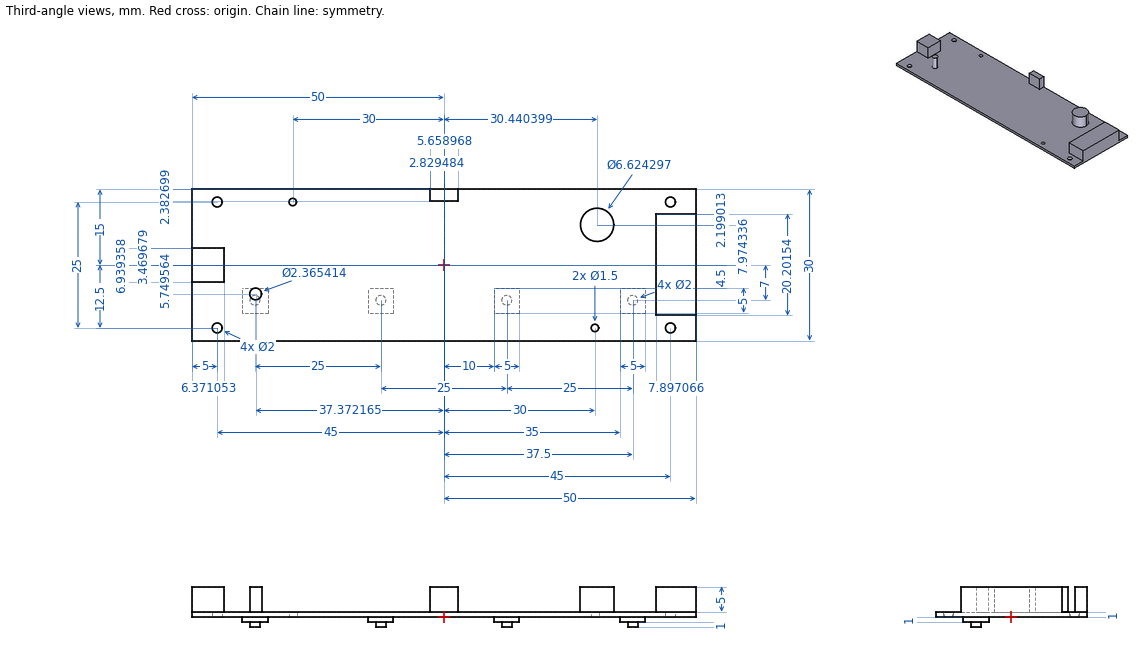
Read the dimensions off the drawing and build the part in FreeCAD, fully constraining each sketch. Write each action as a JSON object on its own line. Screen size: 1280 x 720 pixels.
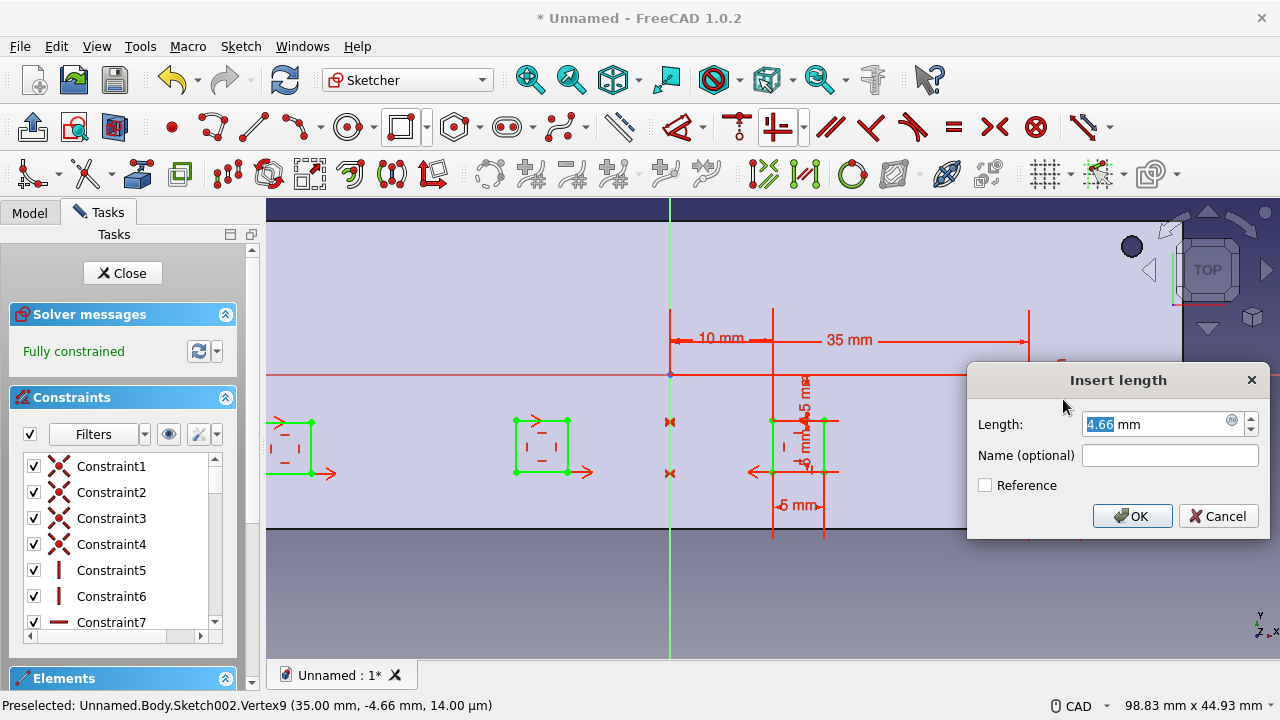
{"action": "type", "text": "4.5"}
{"action": "key", "text": "Return"}
{"action": "key", "text": "Escape"}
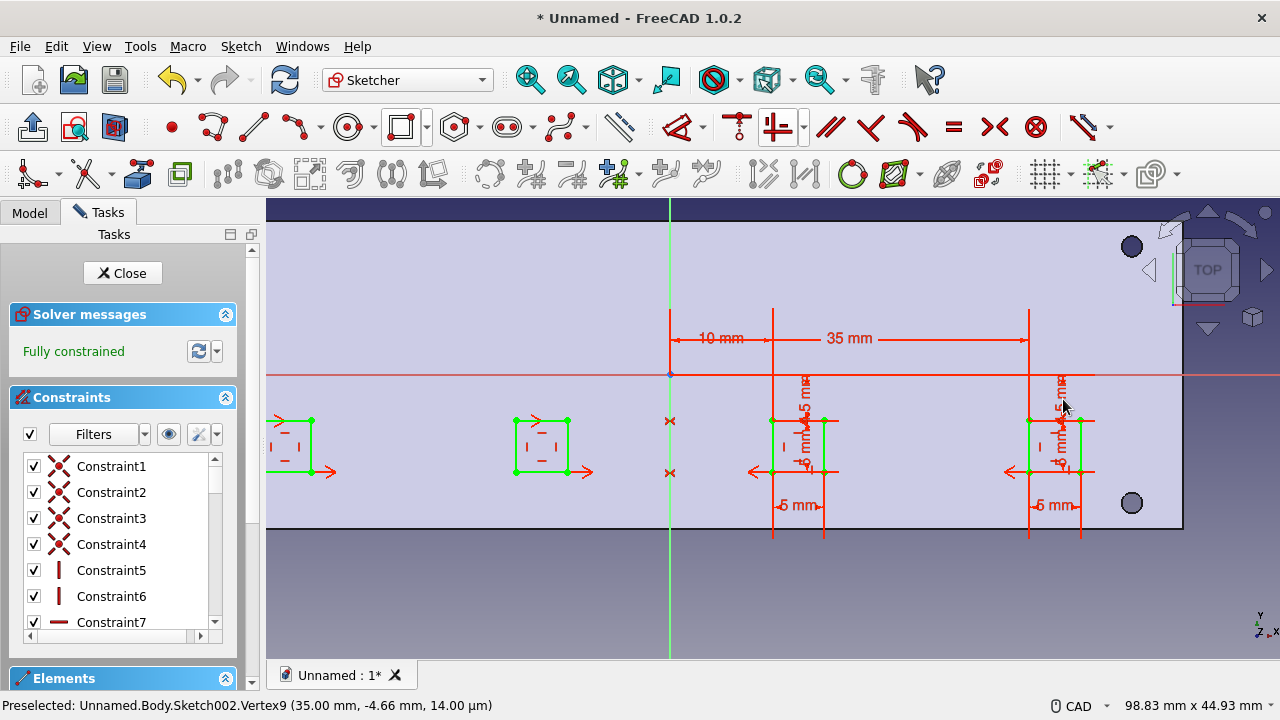
{"action": "left_click", "coordinate": [123, 273]}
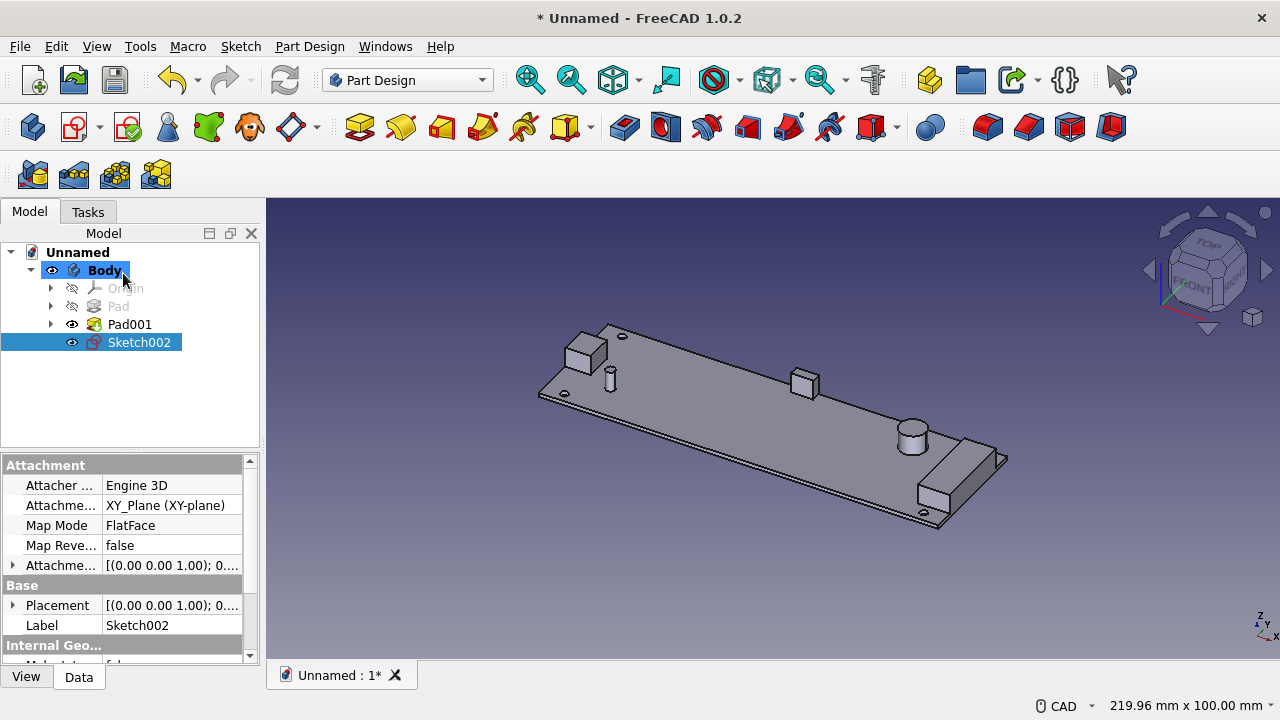
{"action": "left_click", "coordinate": [360, 128]}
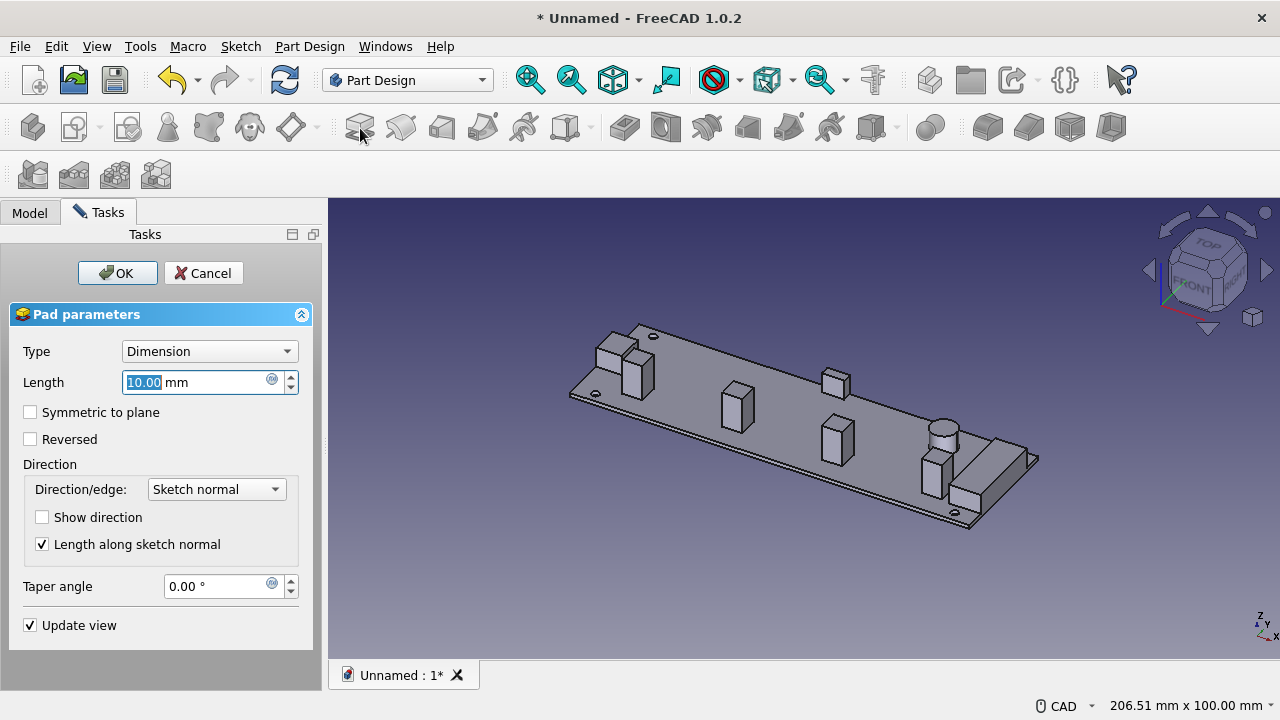
{"action": "type", "text": "1"}
{"action": "key", "text": "Tab"}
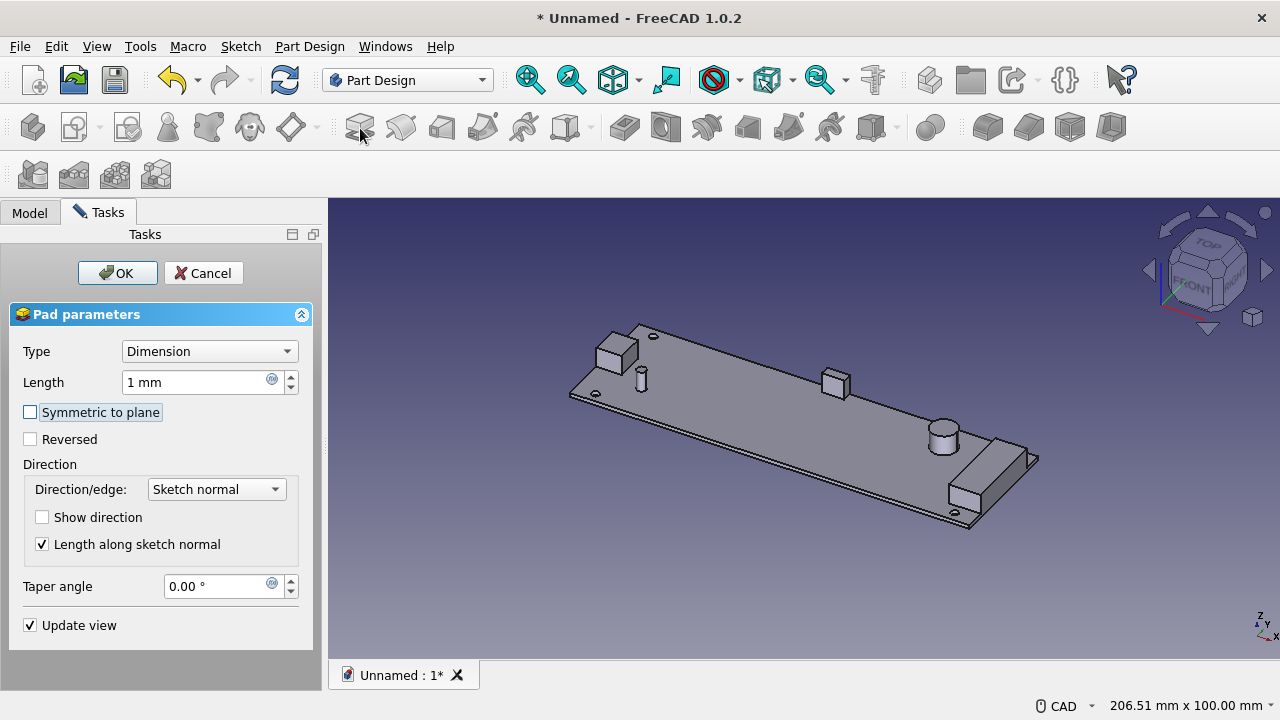
{"action": "left_click", "coordinate": [31, 439]}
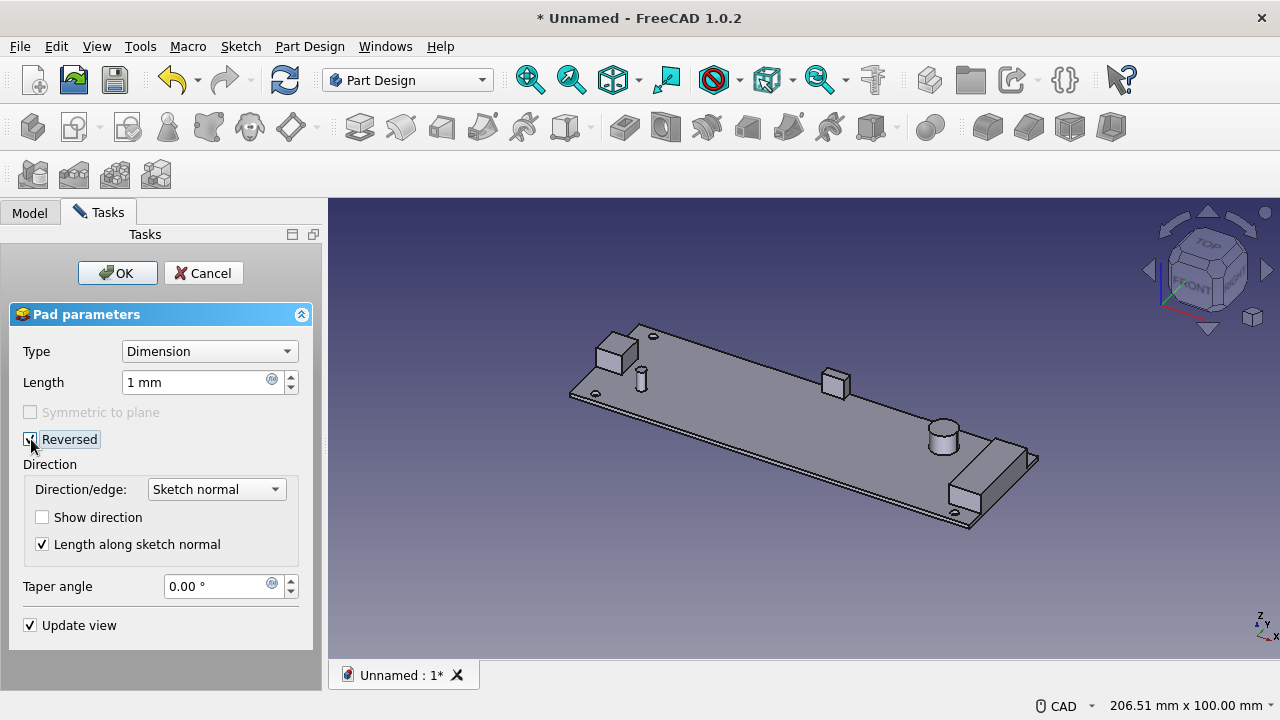
{"action": "left_click", "coordinate": [118, 273]}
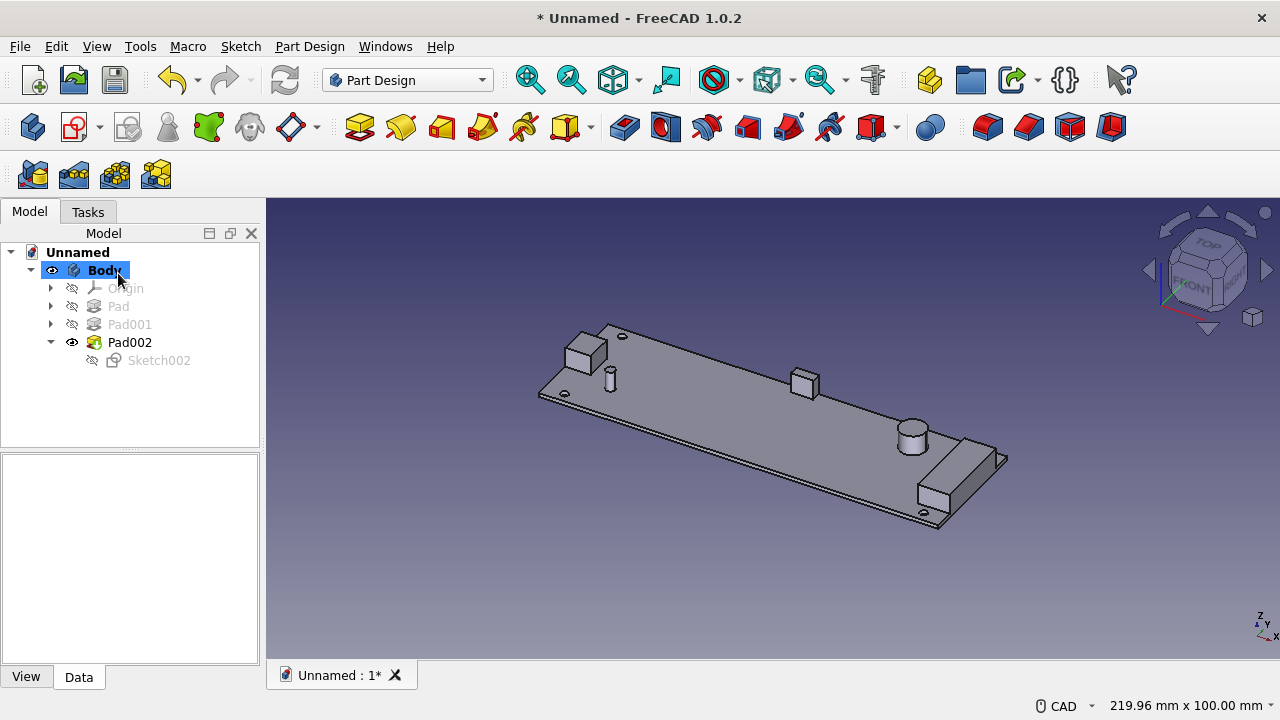
{"action": "key", "text": "5"}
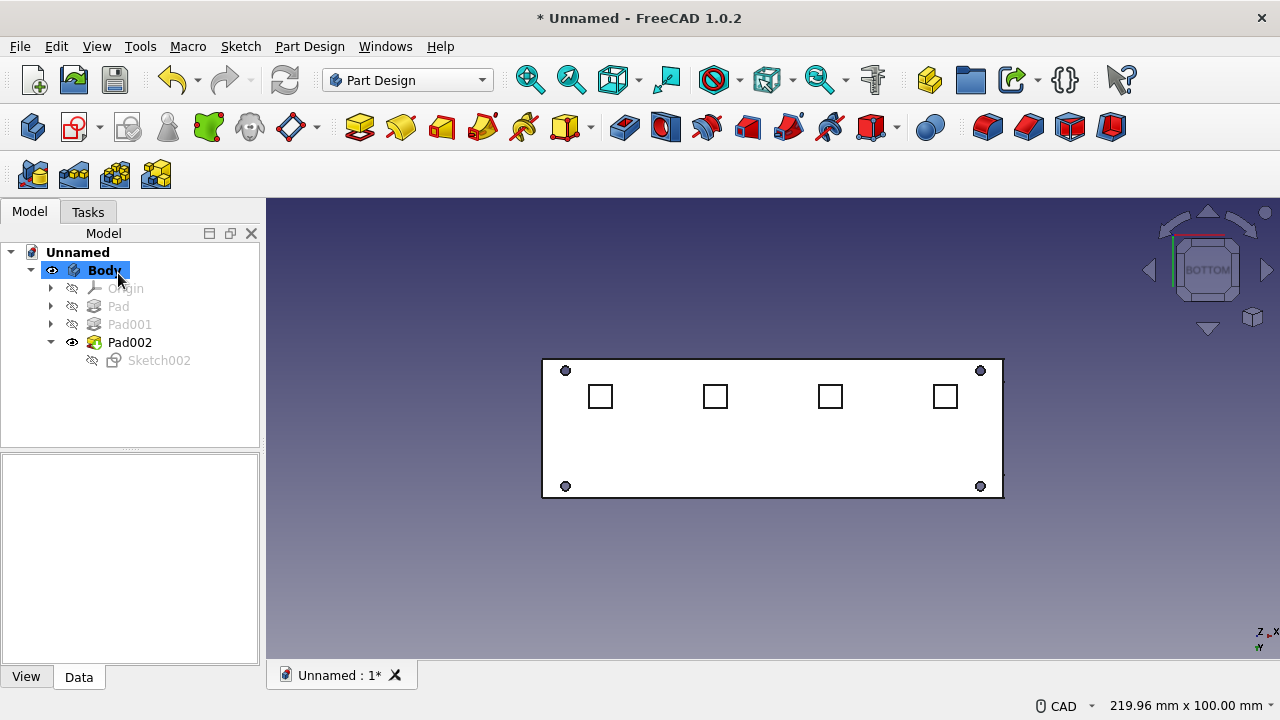
{"action": "left_click", "coordinate": [946, 395]}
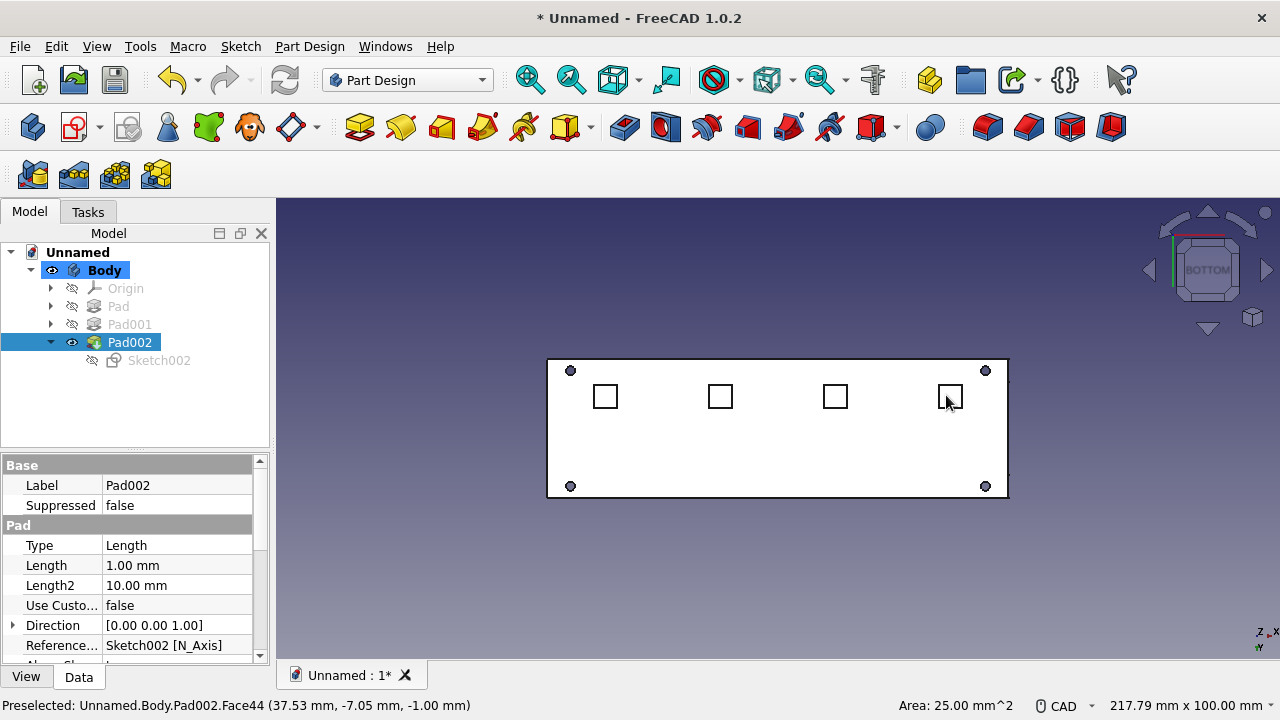
{"action": "left_click", "coordinate": [74, 128]}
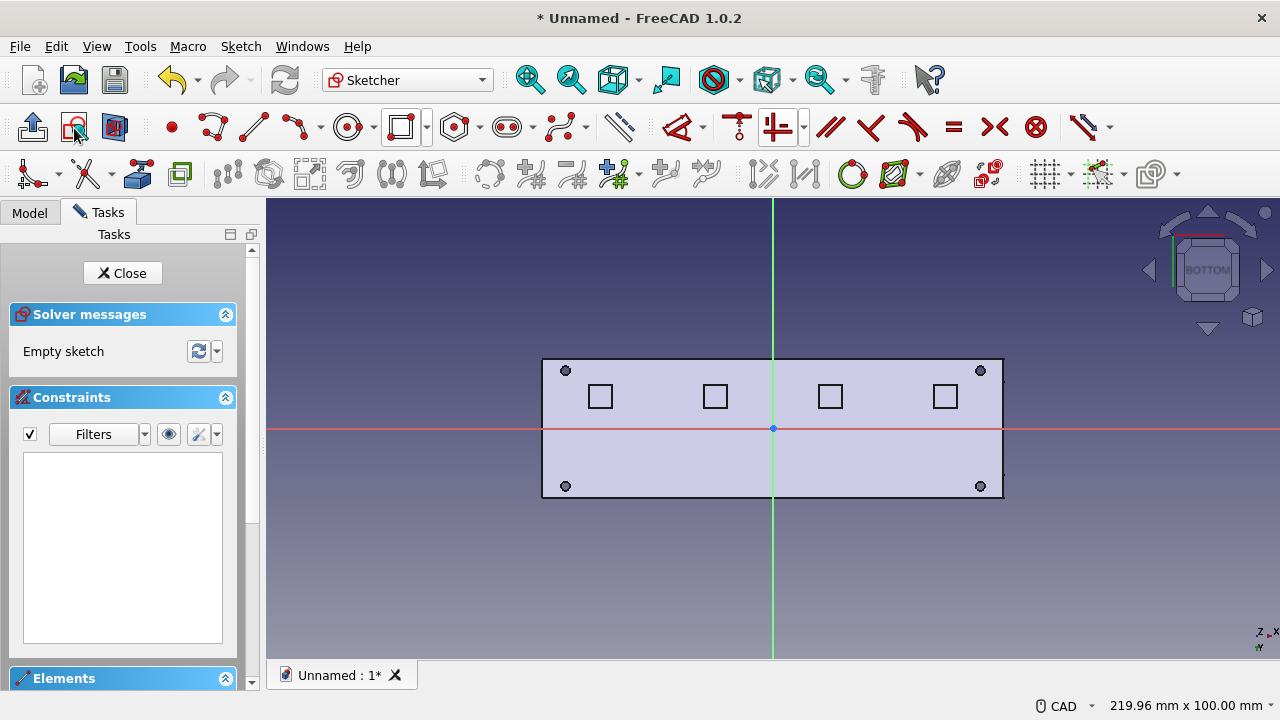
{"action": "scroll", "coordinate": [912, 373], "scroll_direction": "up", "scroll_amount": 2}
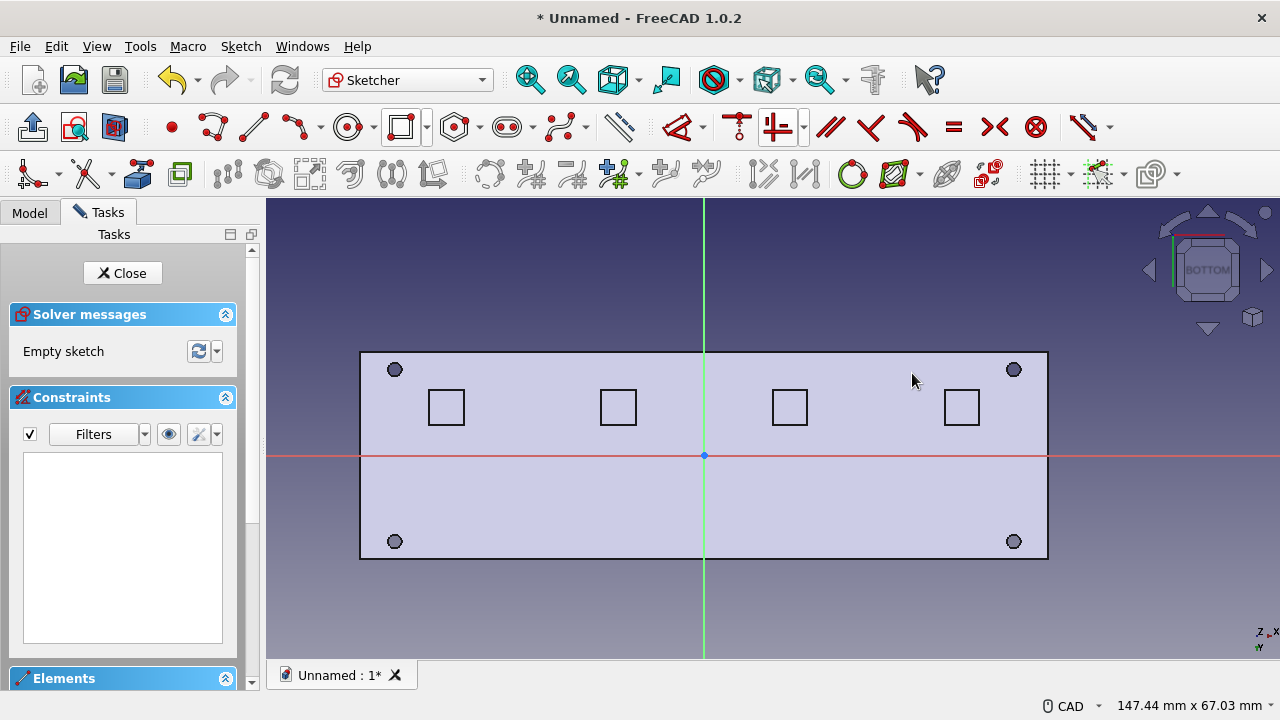
{"action": "left_click", "coordinate": [348, 128]}